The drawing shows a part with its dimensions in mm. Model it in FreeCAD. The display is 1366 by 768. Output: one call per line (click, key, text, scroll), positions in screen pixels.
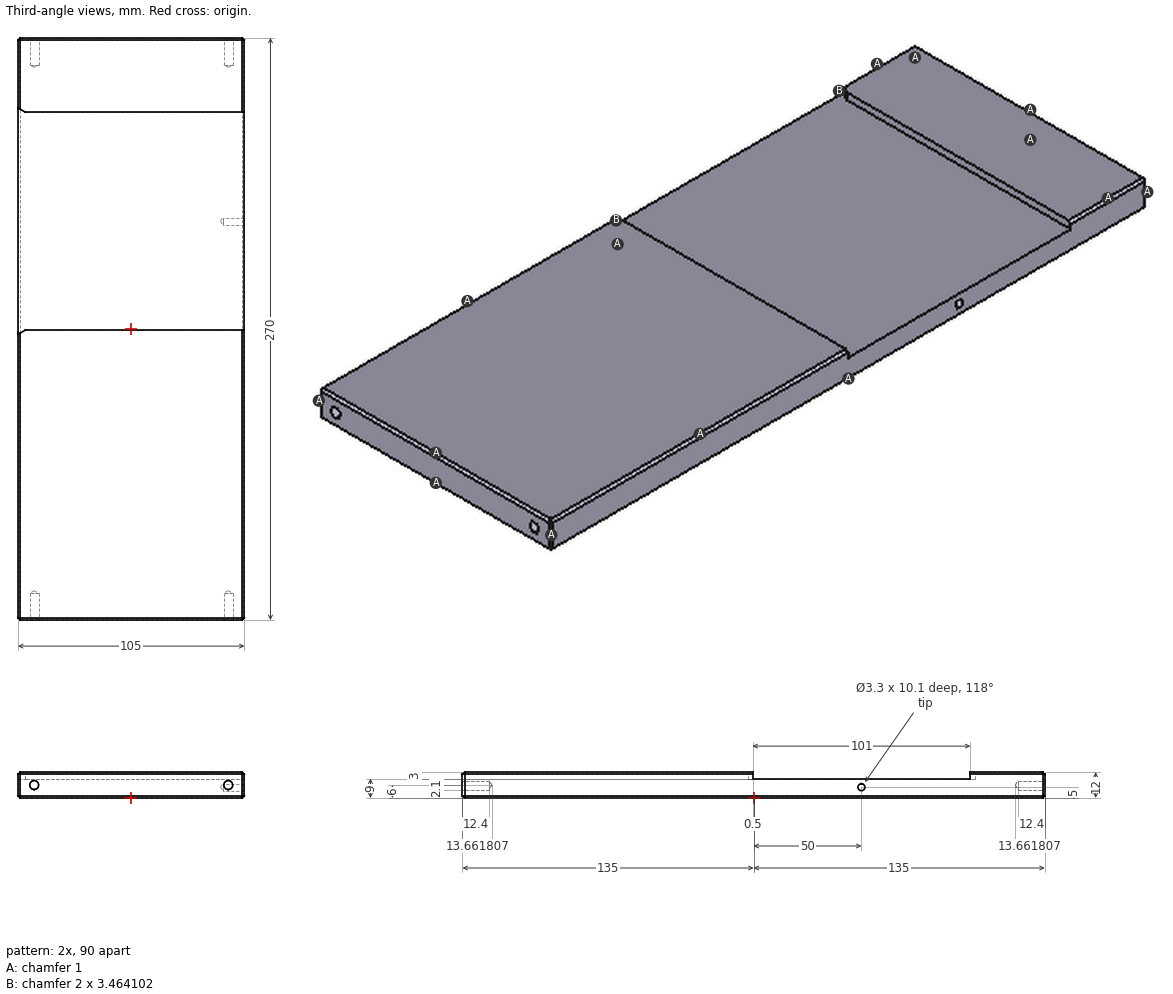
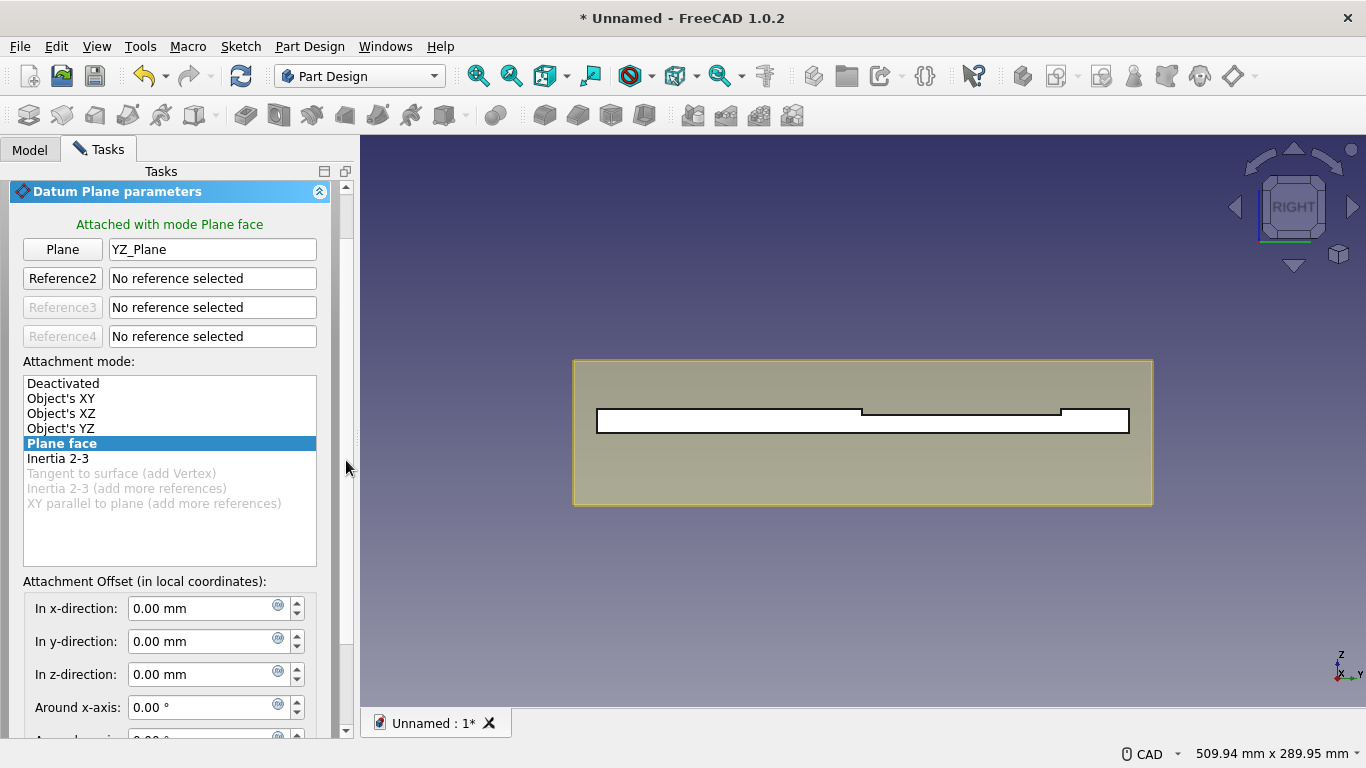
triple_click(210, 614)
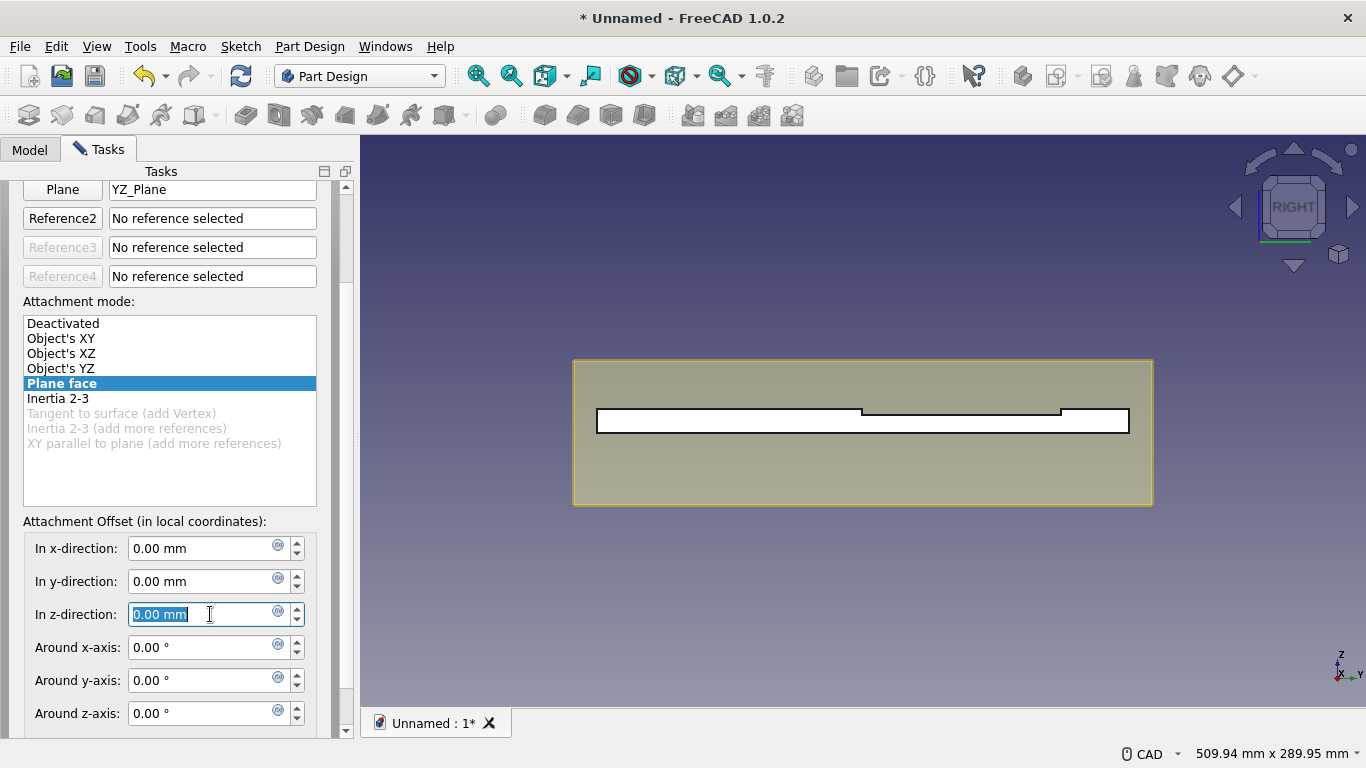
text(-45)
key(Tab)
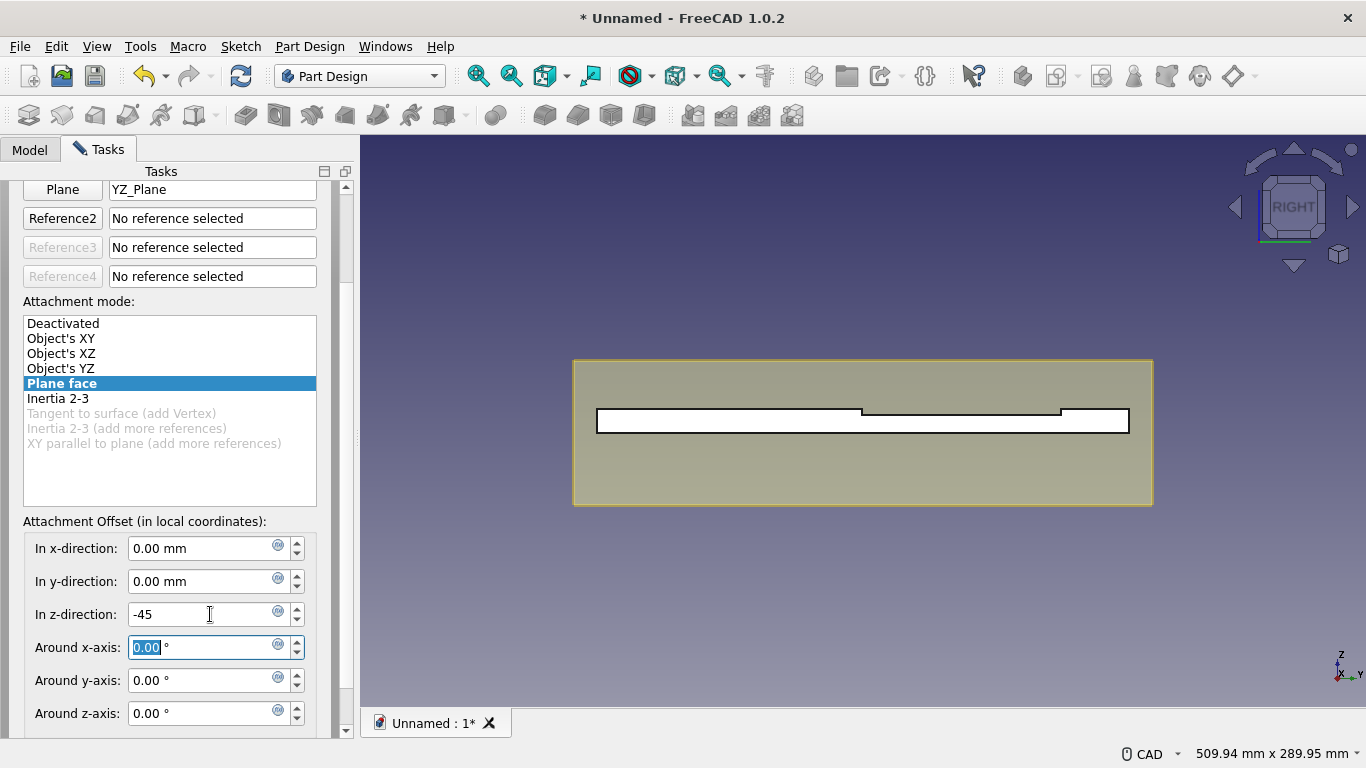
scroll(346, 460, up, 3)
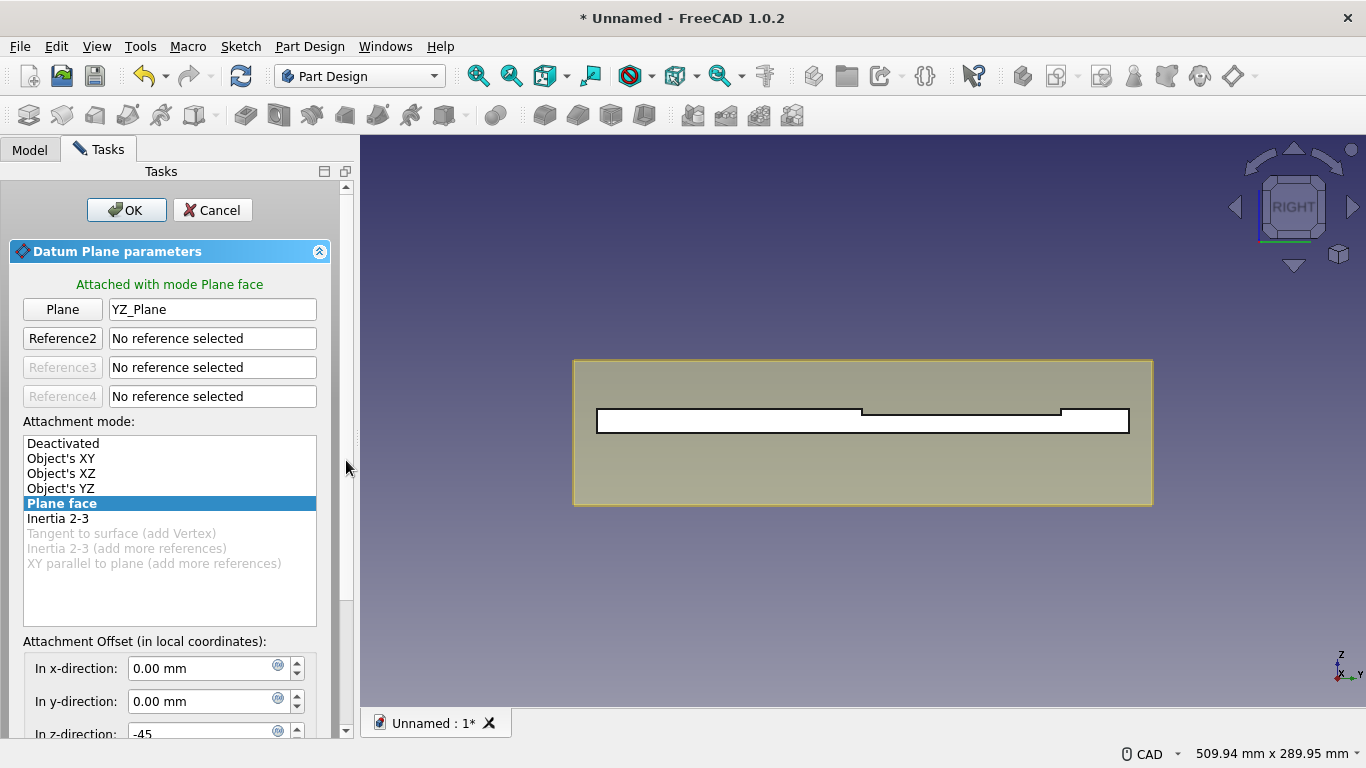
click(127, 210)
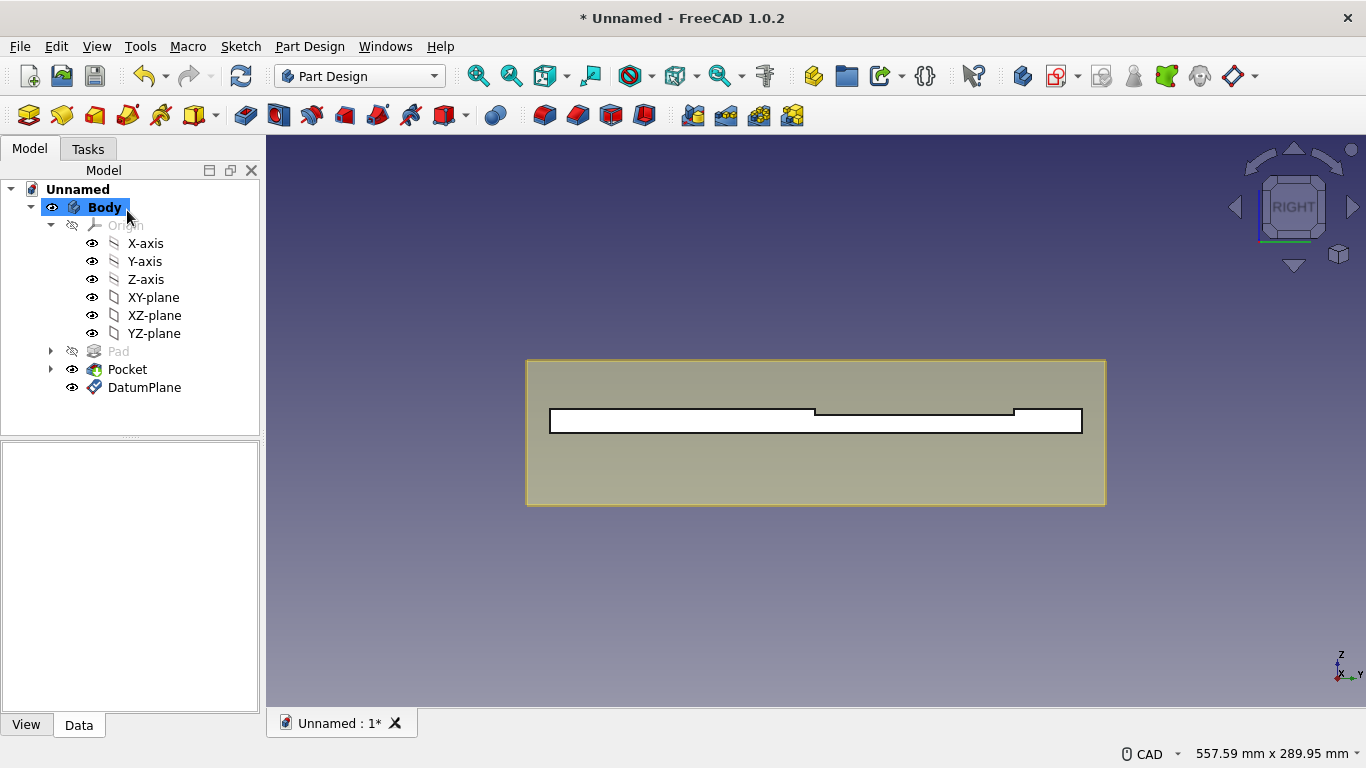
click(117, 387)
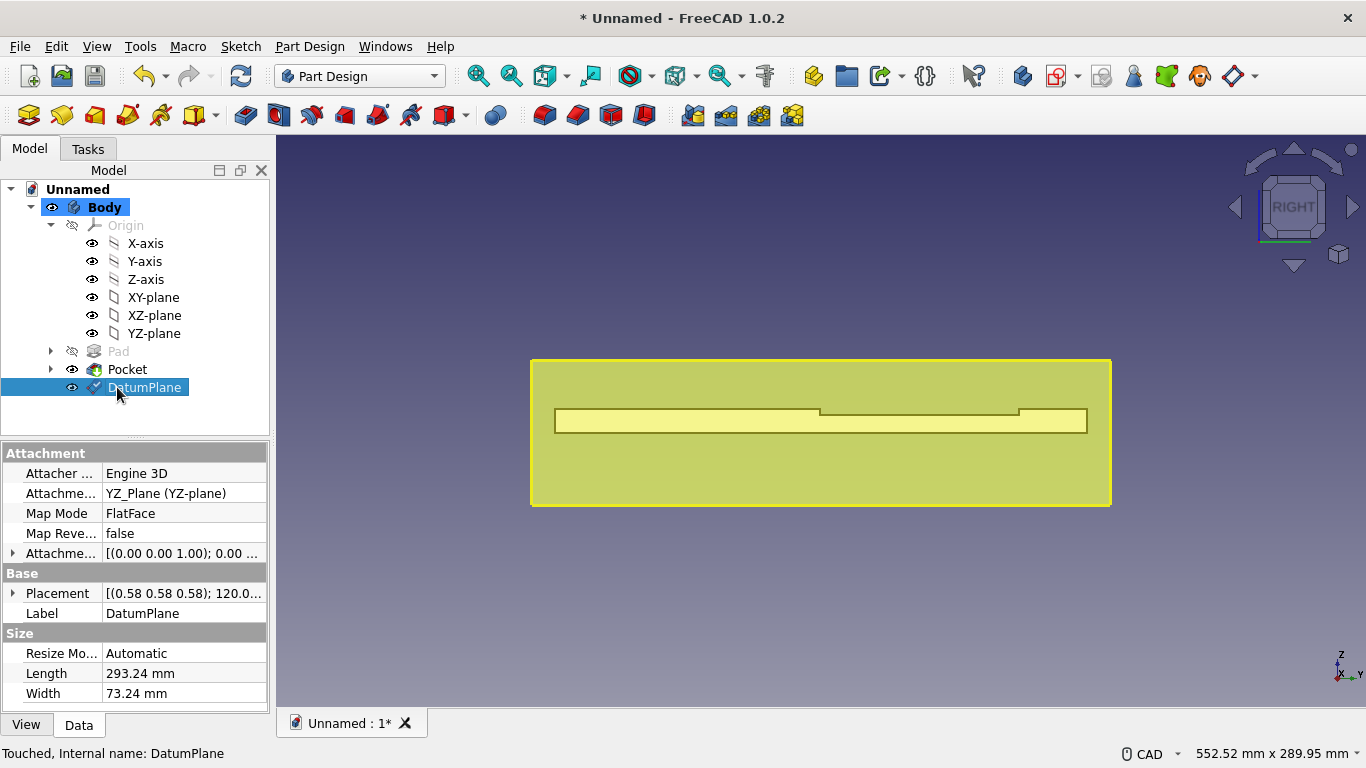
click(1056, 76)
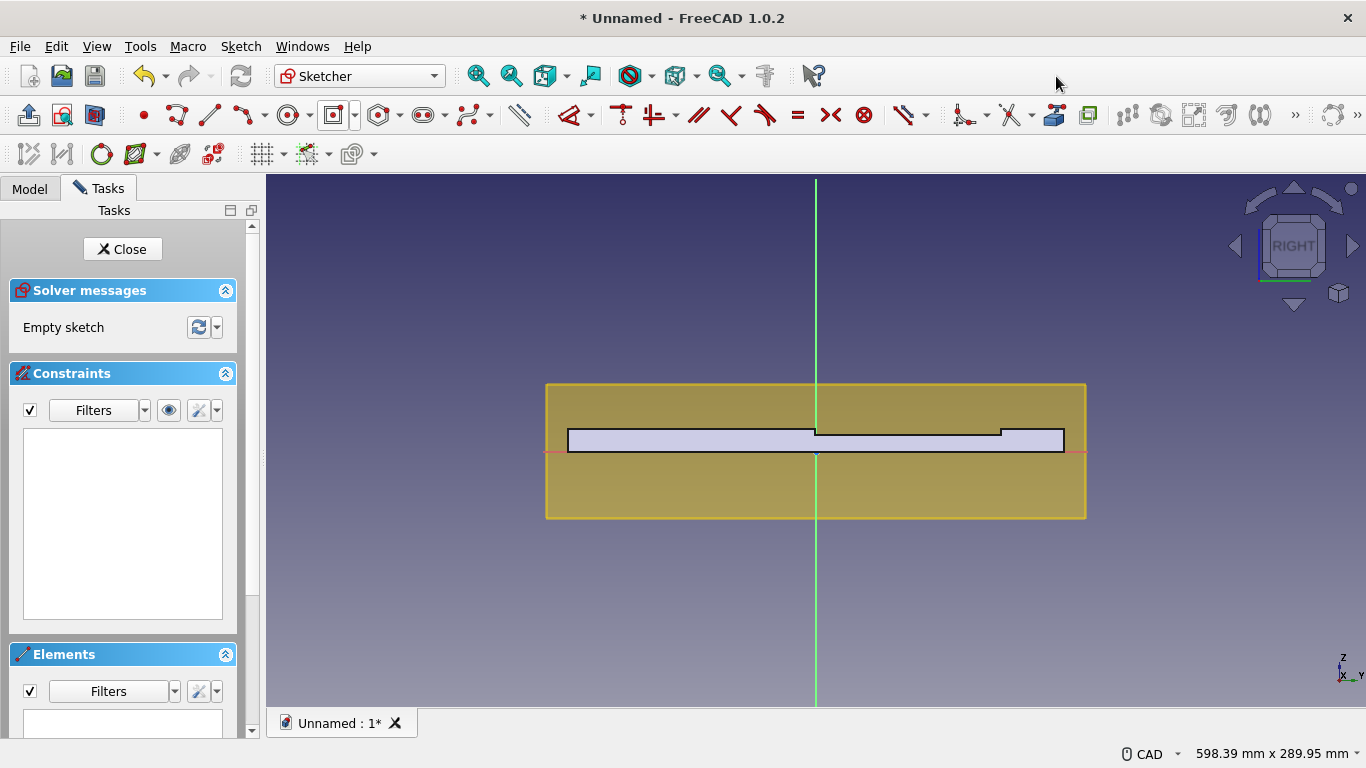
click(95, 116)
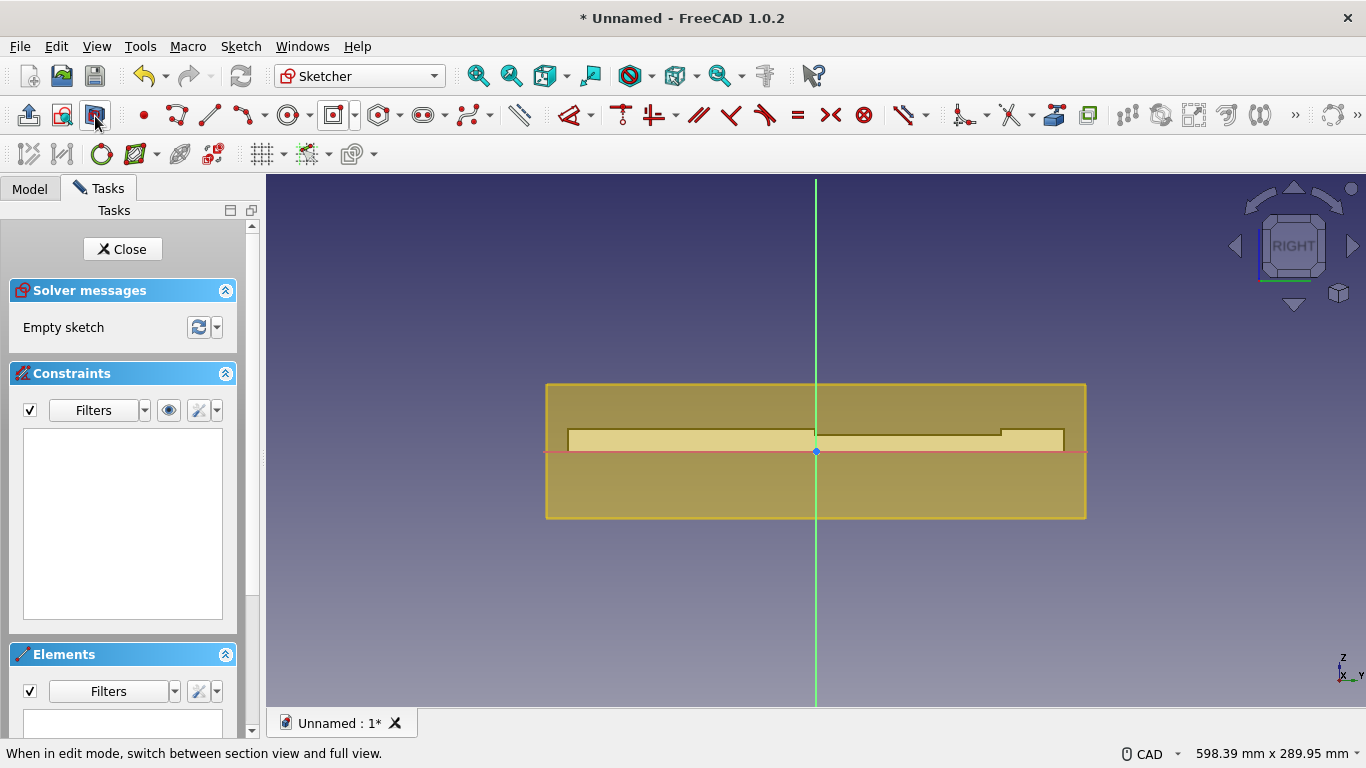
scroll(577, 443, up, 15)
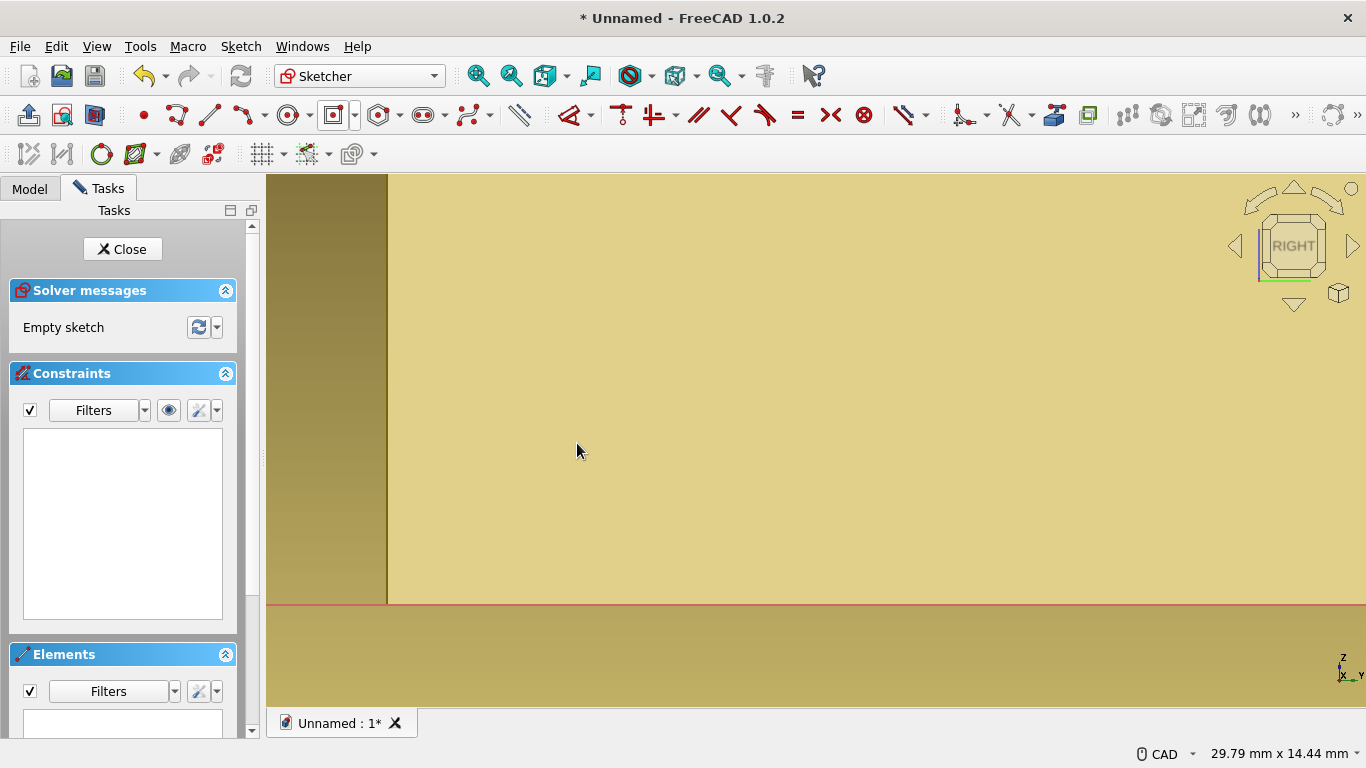
click(177, 116)